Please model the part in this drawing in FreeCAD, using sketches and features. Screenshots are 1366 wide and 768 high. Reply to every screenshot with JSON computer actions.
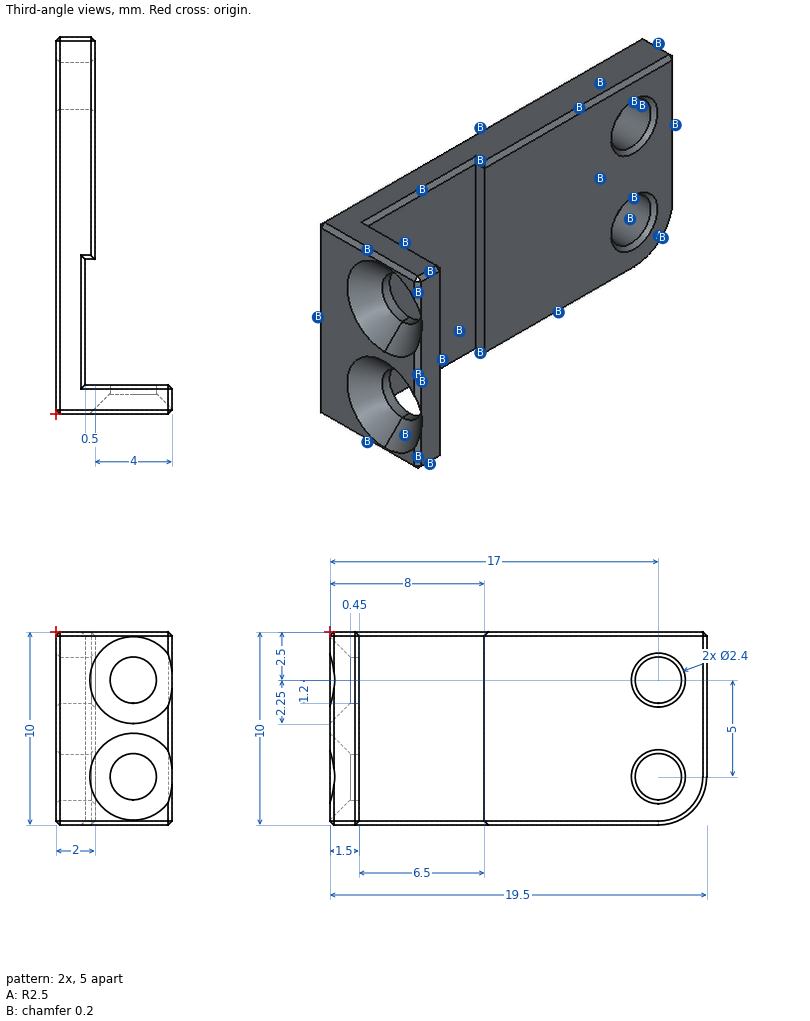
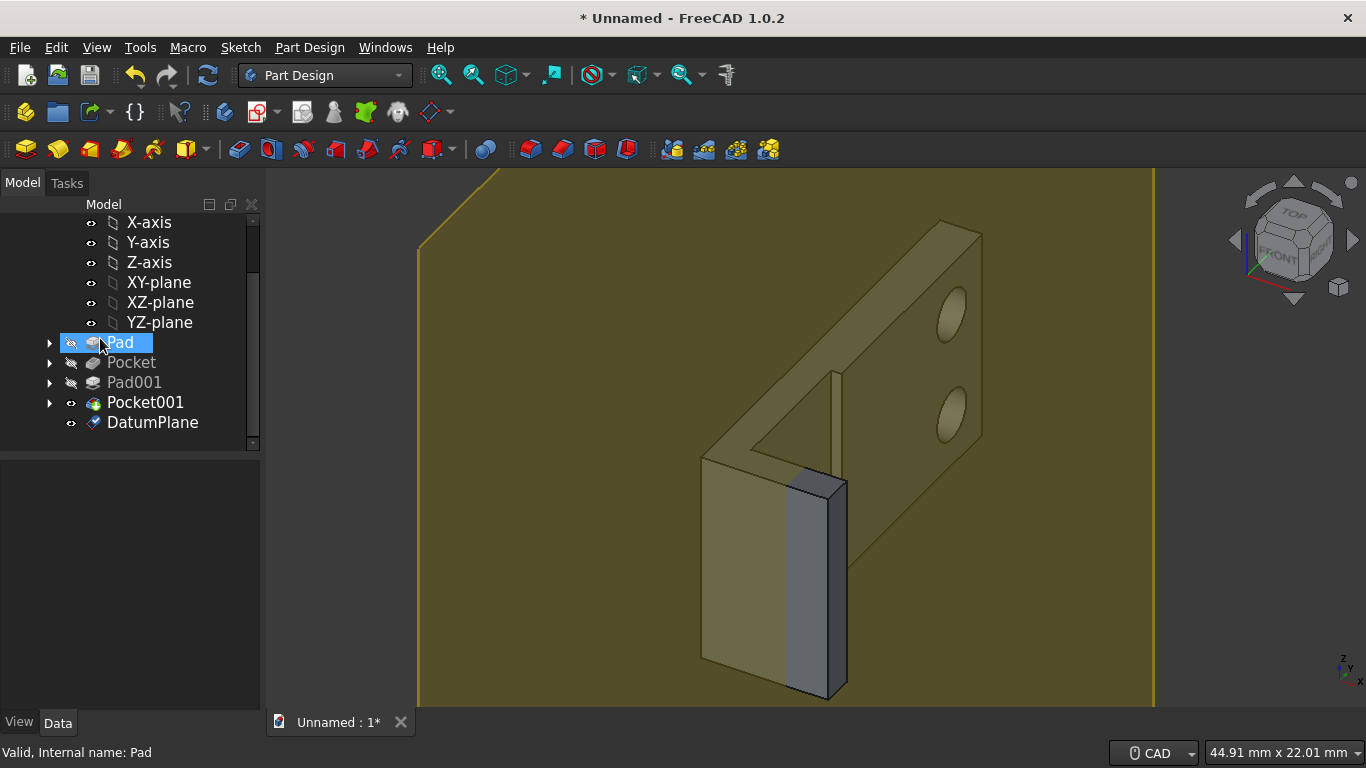
{"action": "left_click", "coordinate": [116, 423]}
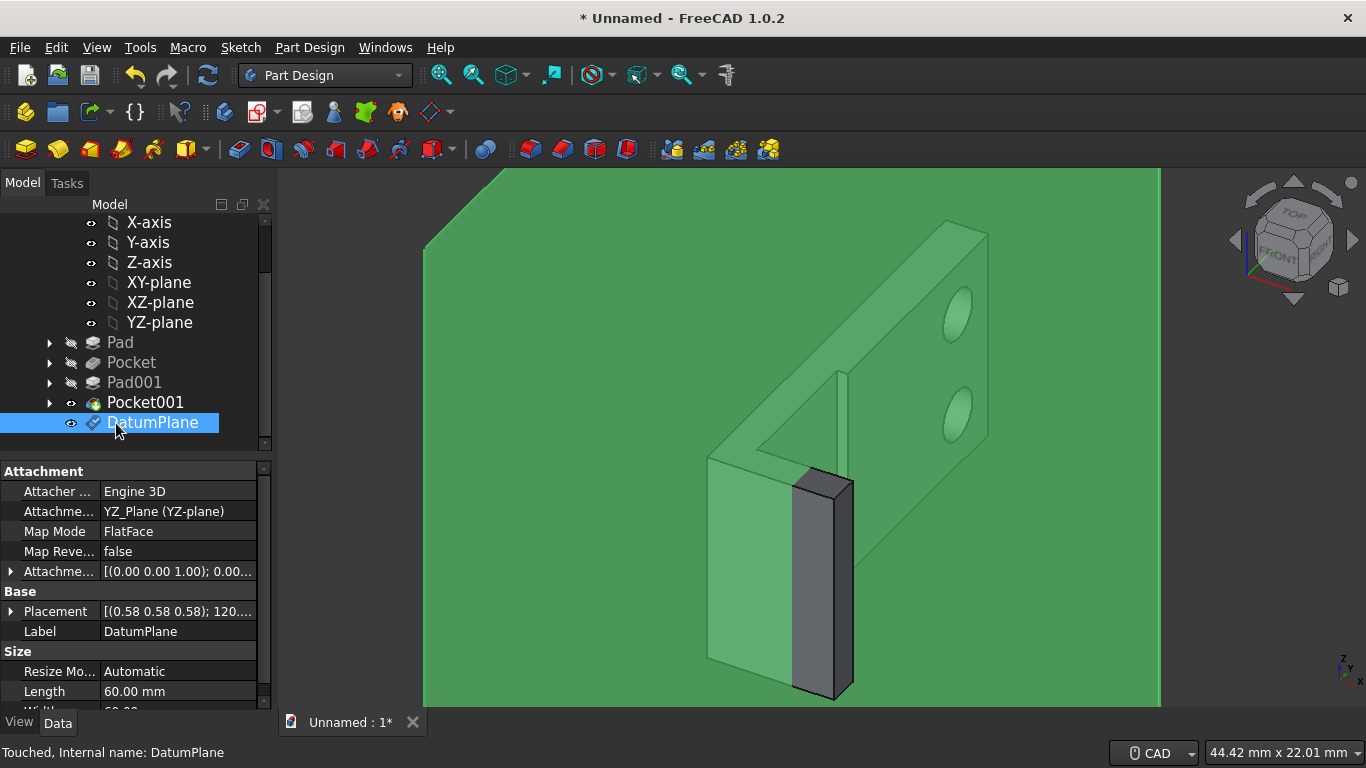
{"action": "left_click", "coordinate": [258, 112]}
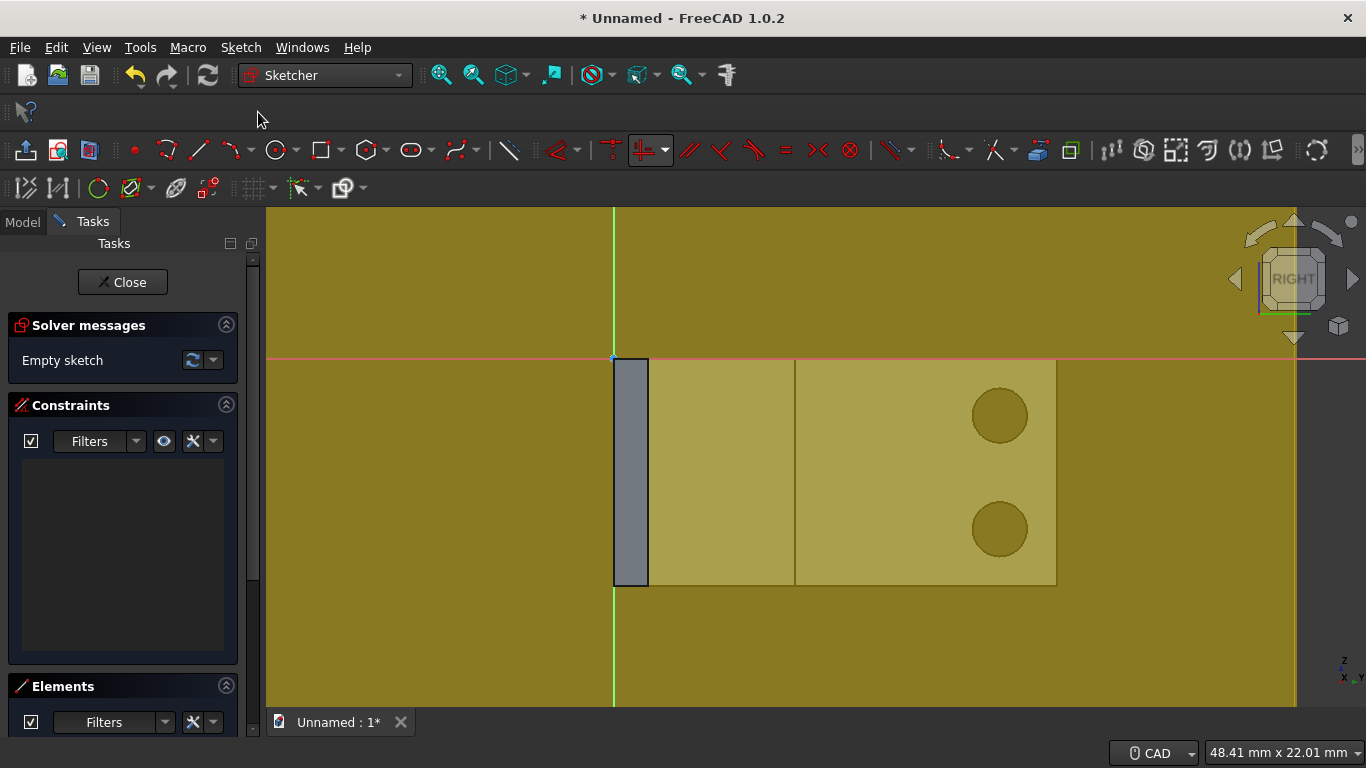
{"action": "left_click", "coordinate": [90, 150]}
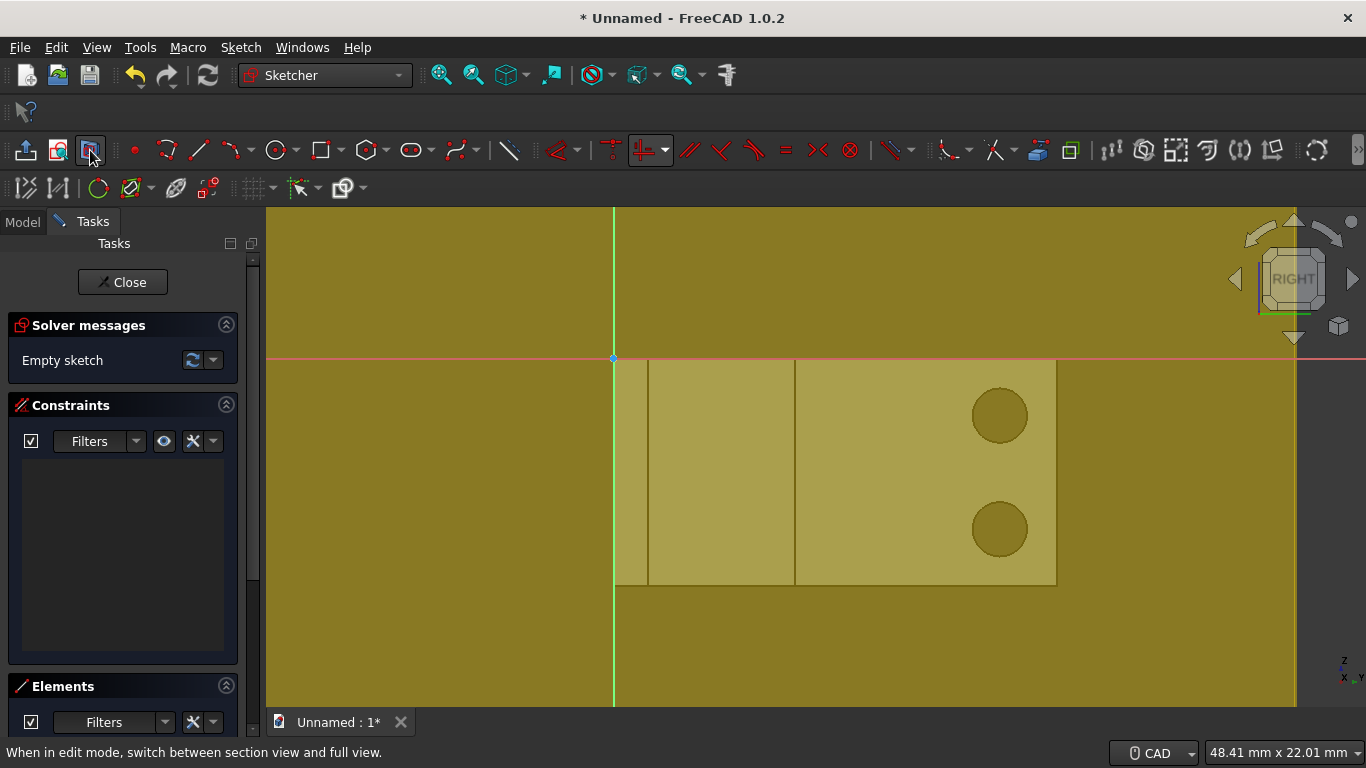
{"action": "scroll", "coordinate": [573, 387], "scroll_direction": "up", "scroll_amount": 5}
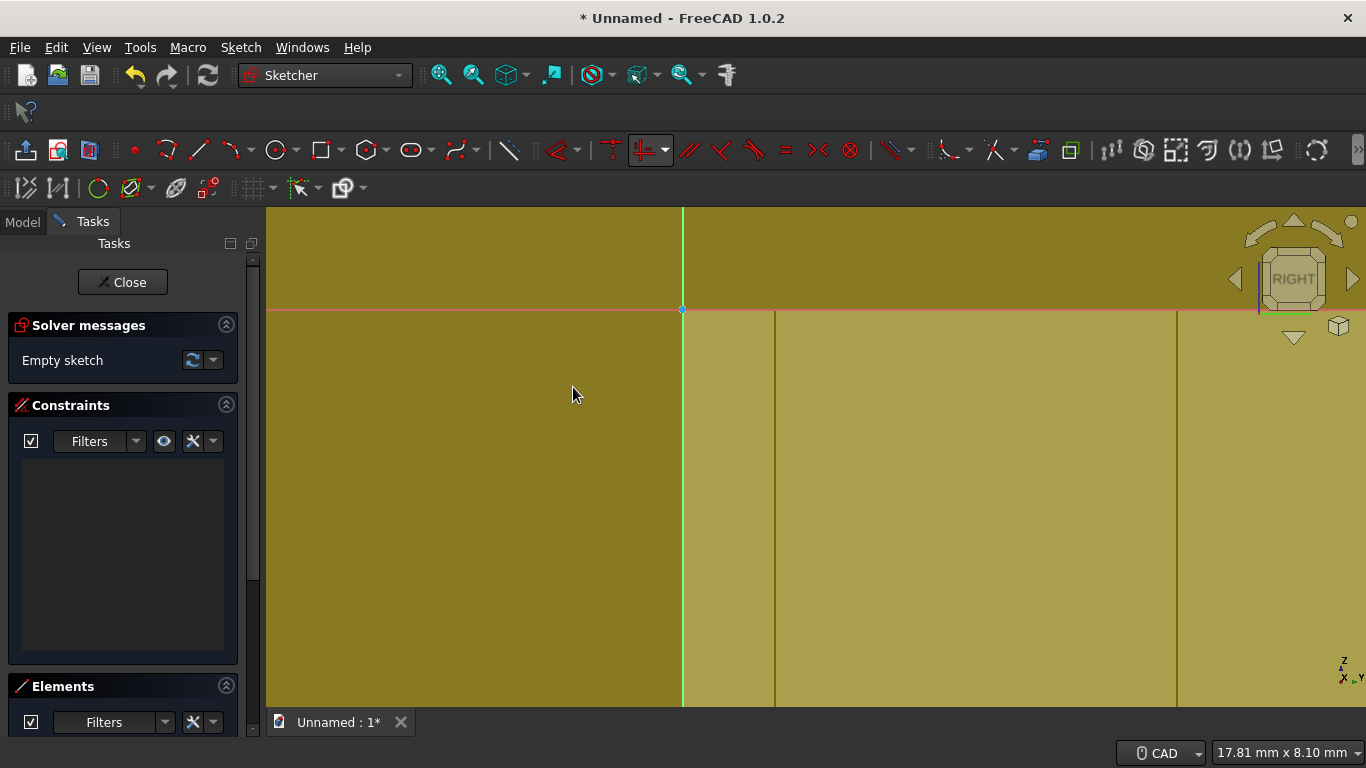
{"action": "left_click", "coordinate": [168, 150]}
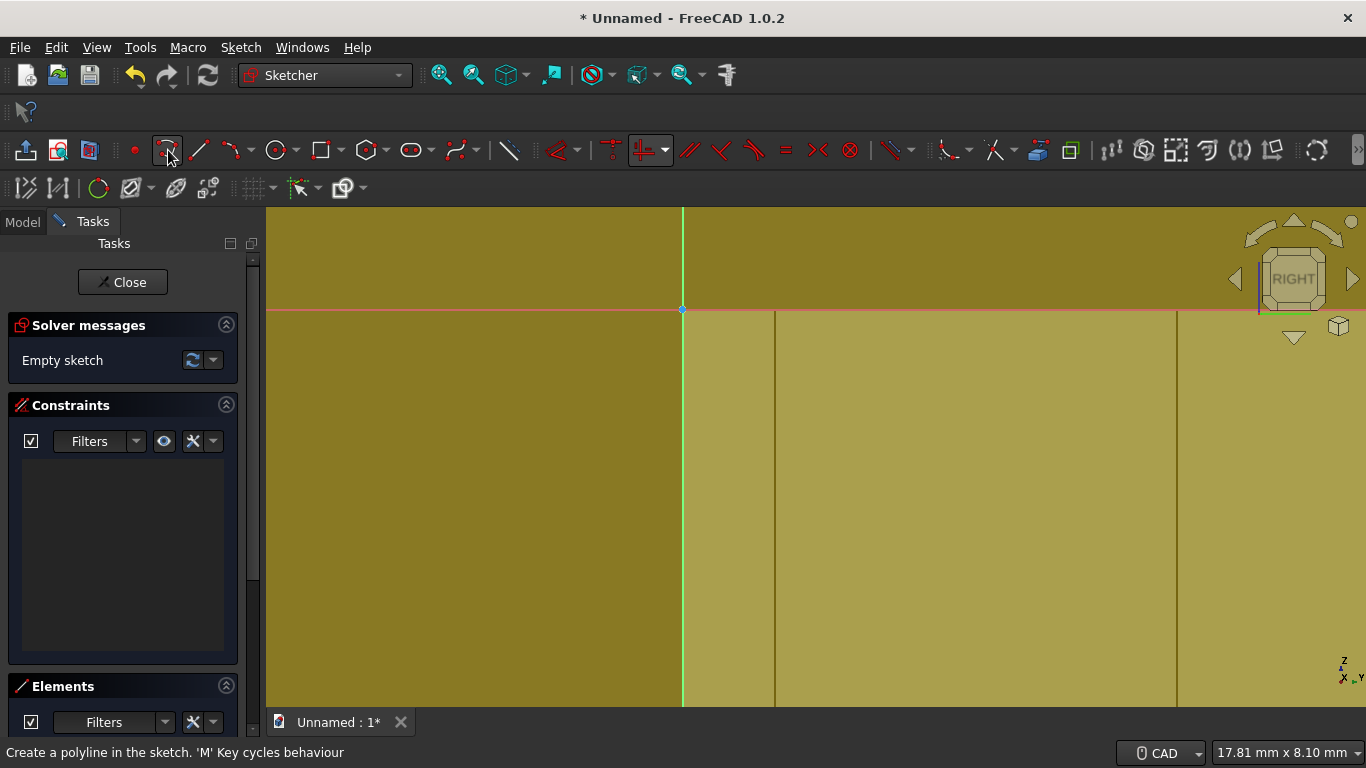
{"action": "left_click", "coordinate": [683, 464]}
{"action": "left_click", "coordinate": [692, 603]}
{"action": "left_click", "coordinate": [748, 538]}
{"action": "left_click", "coordinate": [775, 538]}
{"action": "left_click", "coordinate": [775, 464]}
{"action": "left_click", "coordinate": [683, 465]}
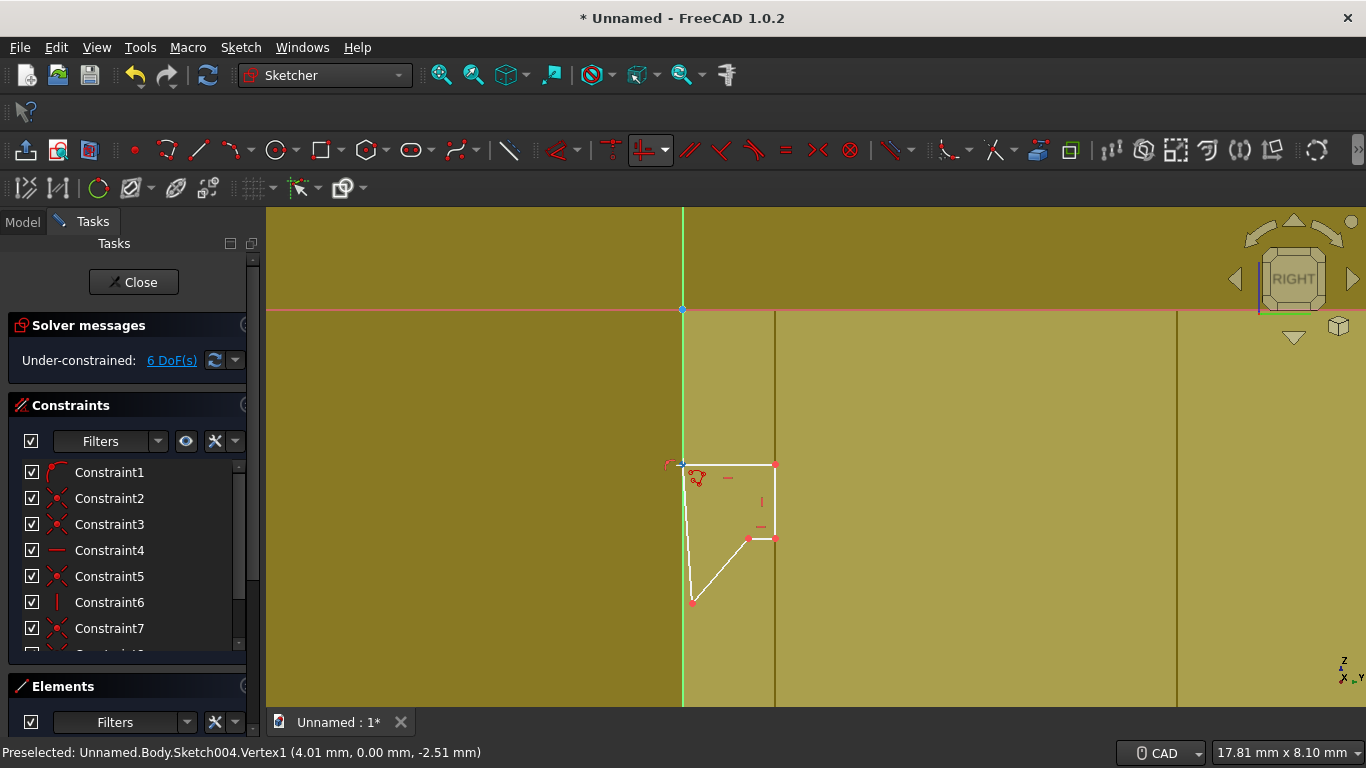
{"action": "left_click", "coordinate": [200, 150]}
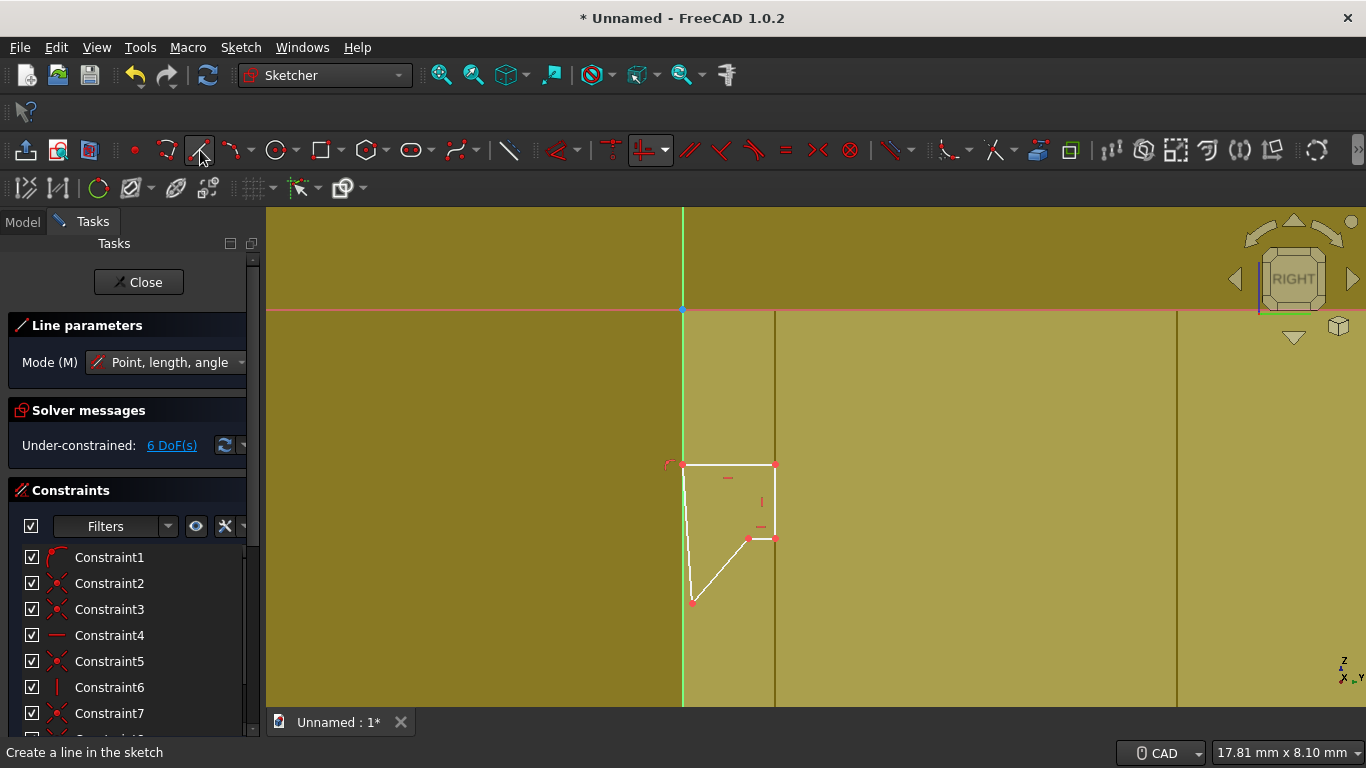
{"action": "scroll", "coordinate": [785, 464], "scroll_direction": "up", "scroll_amount": 3}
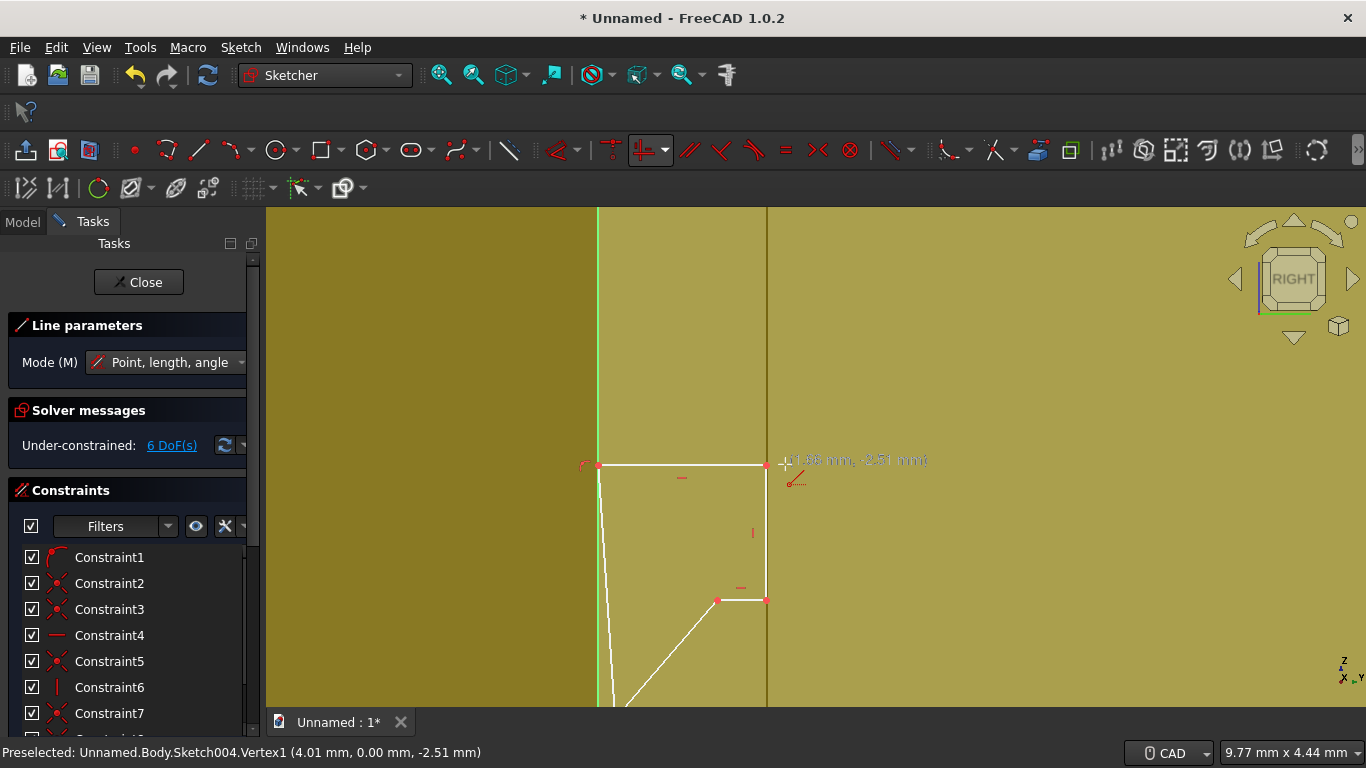
{"action": "left_click", "coordinate": [784, 464]}
{"action": "left_click", "coordinate": [835, 464]}
{"action": "key", "text": "Escape"}